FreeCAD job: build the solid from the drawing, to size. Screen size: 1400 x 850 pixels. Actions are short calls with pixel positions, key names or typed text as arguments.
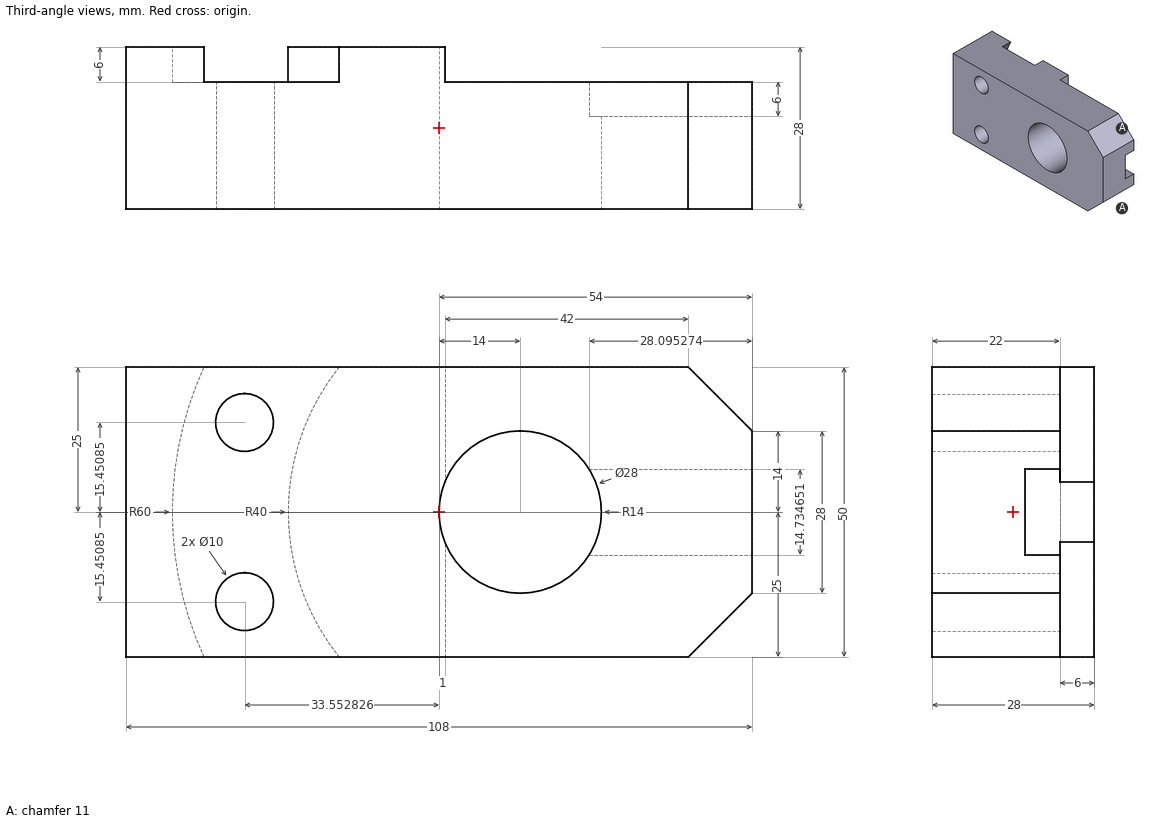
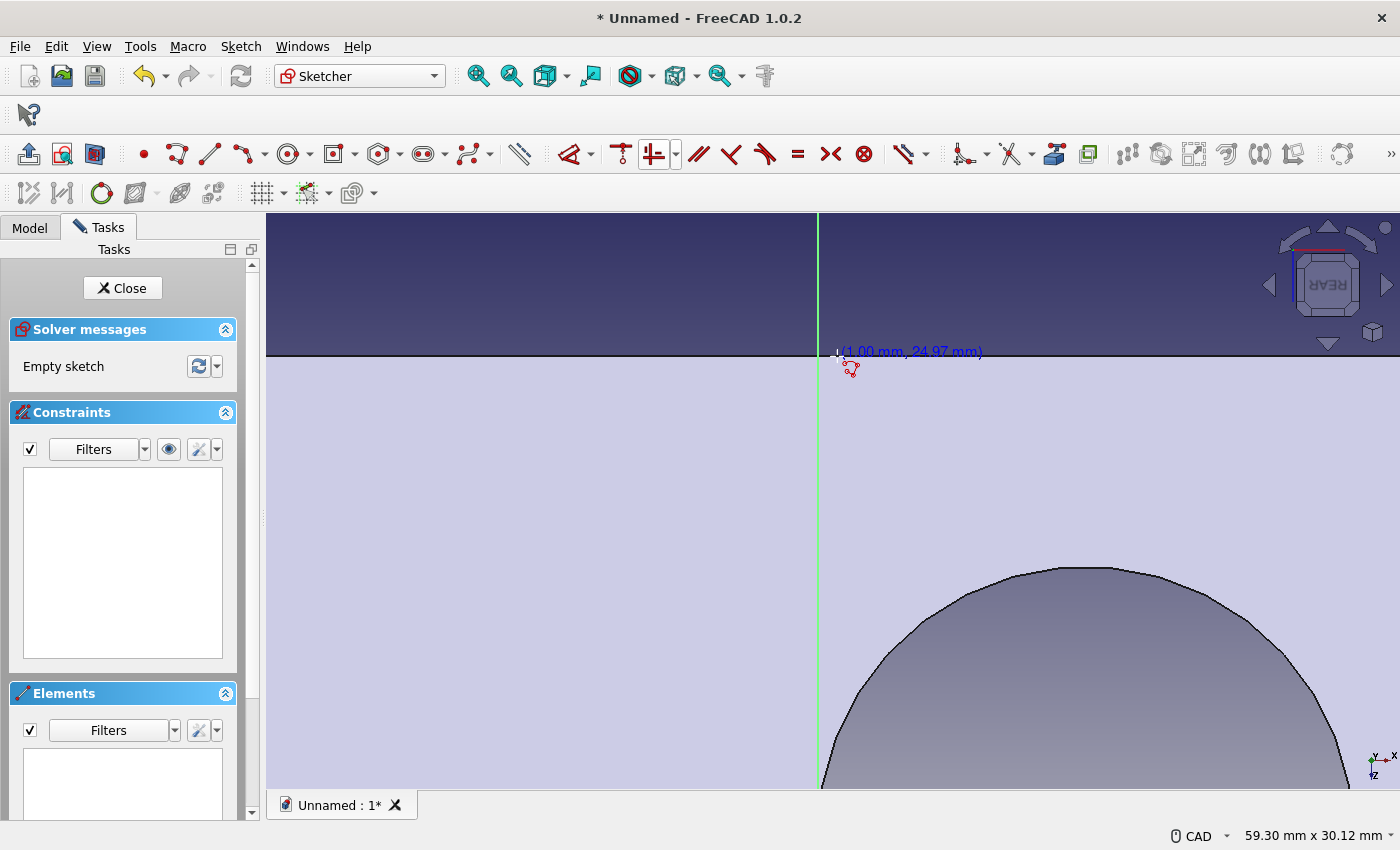
scroll(433, 307, down, 5)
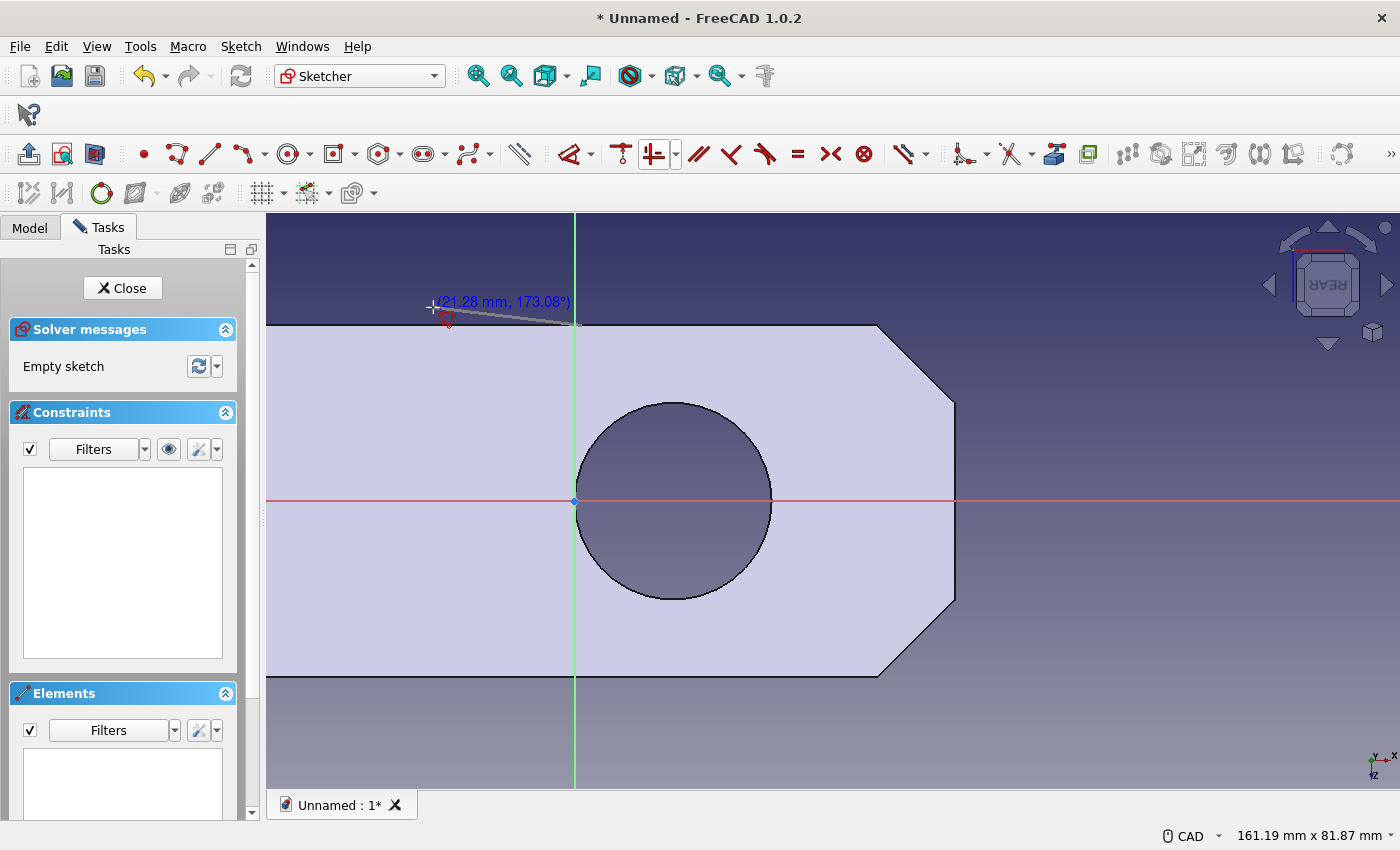
scroll(582, 677, up, 5)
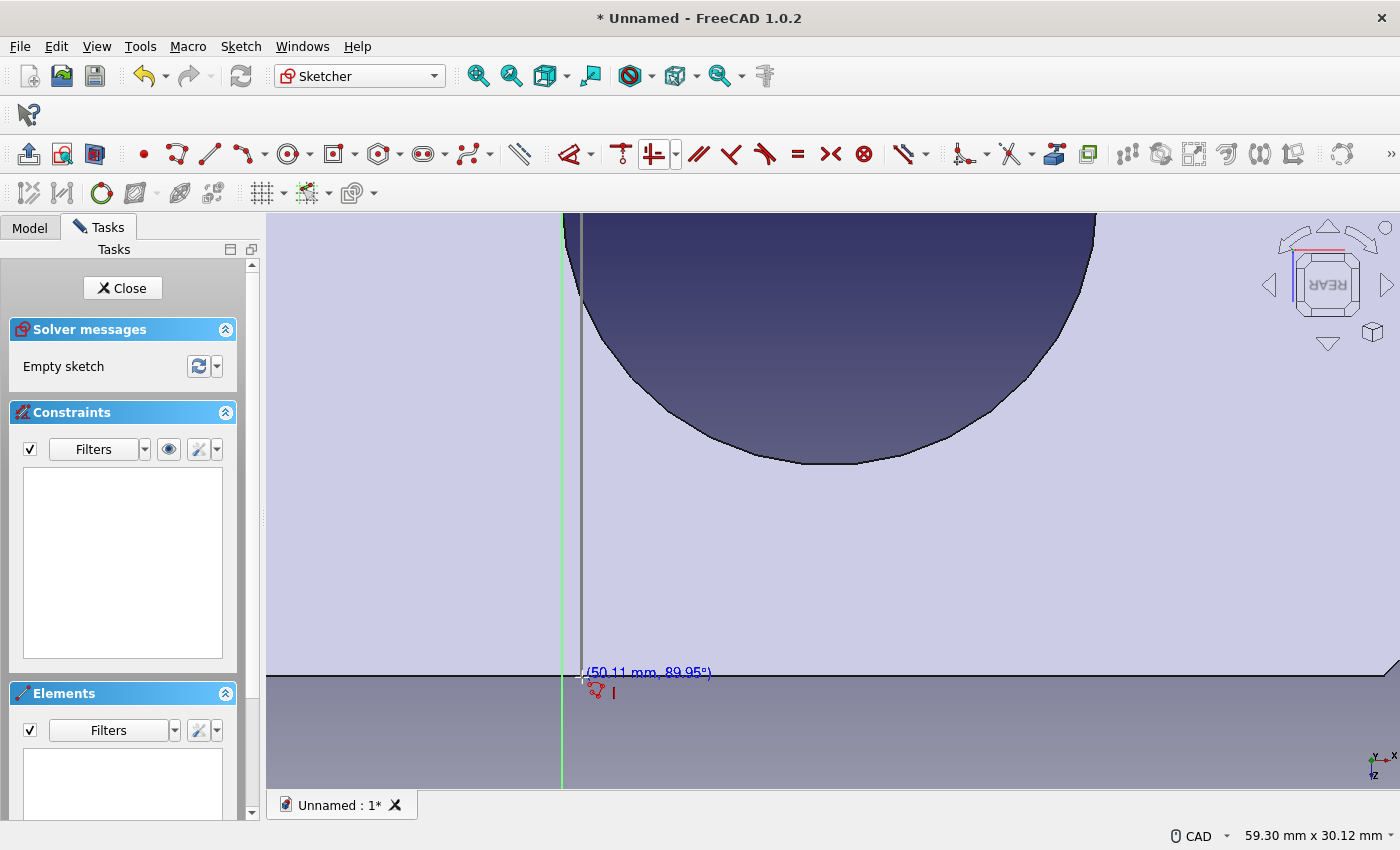
click(581, 676)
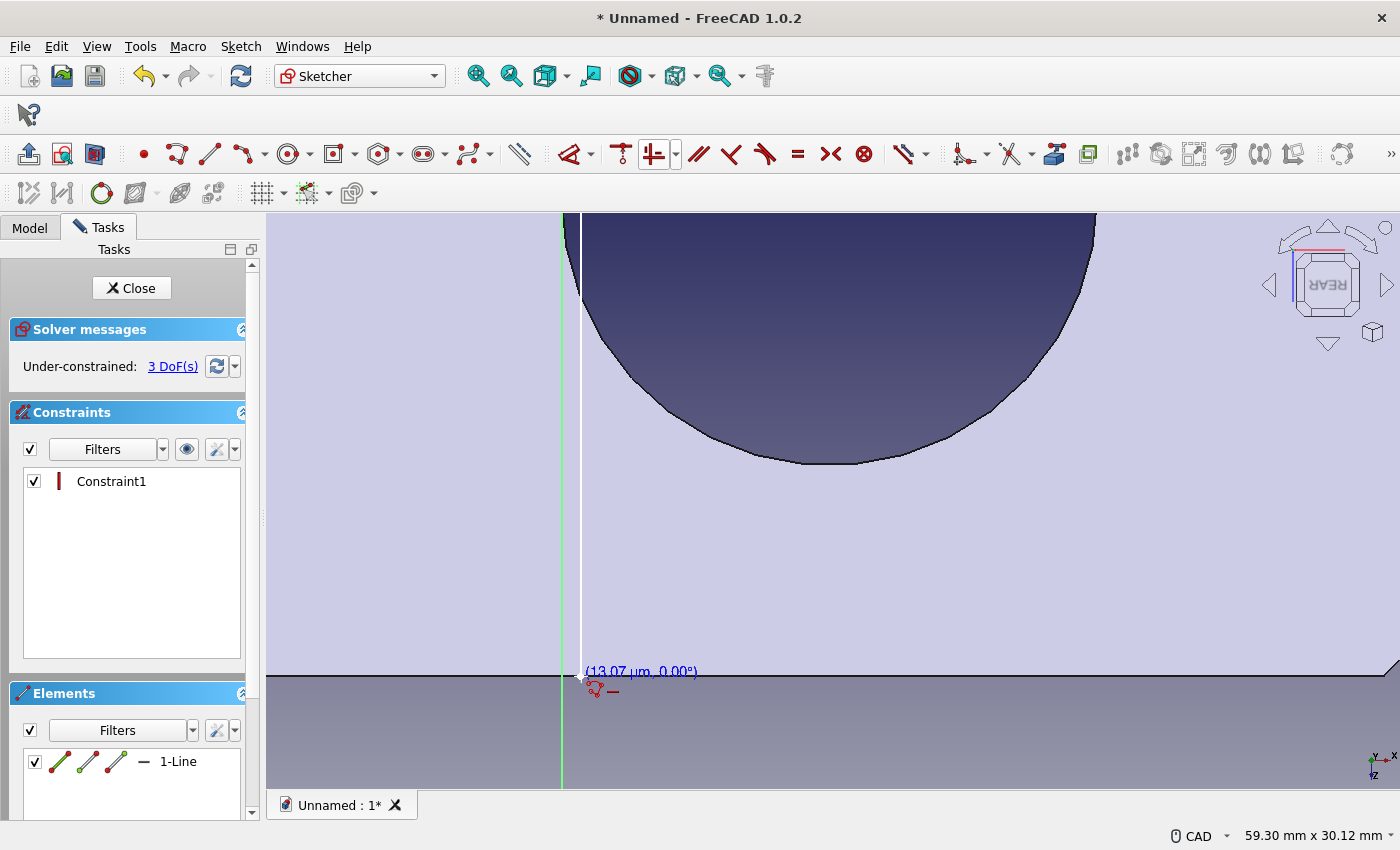
scroll(582, 678, down, 5)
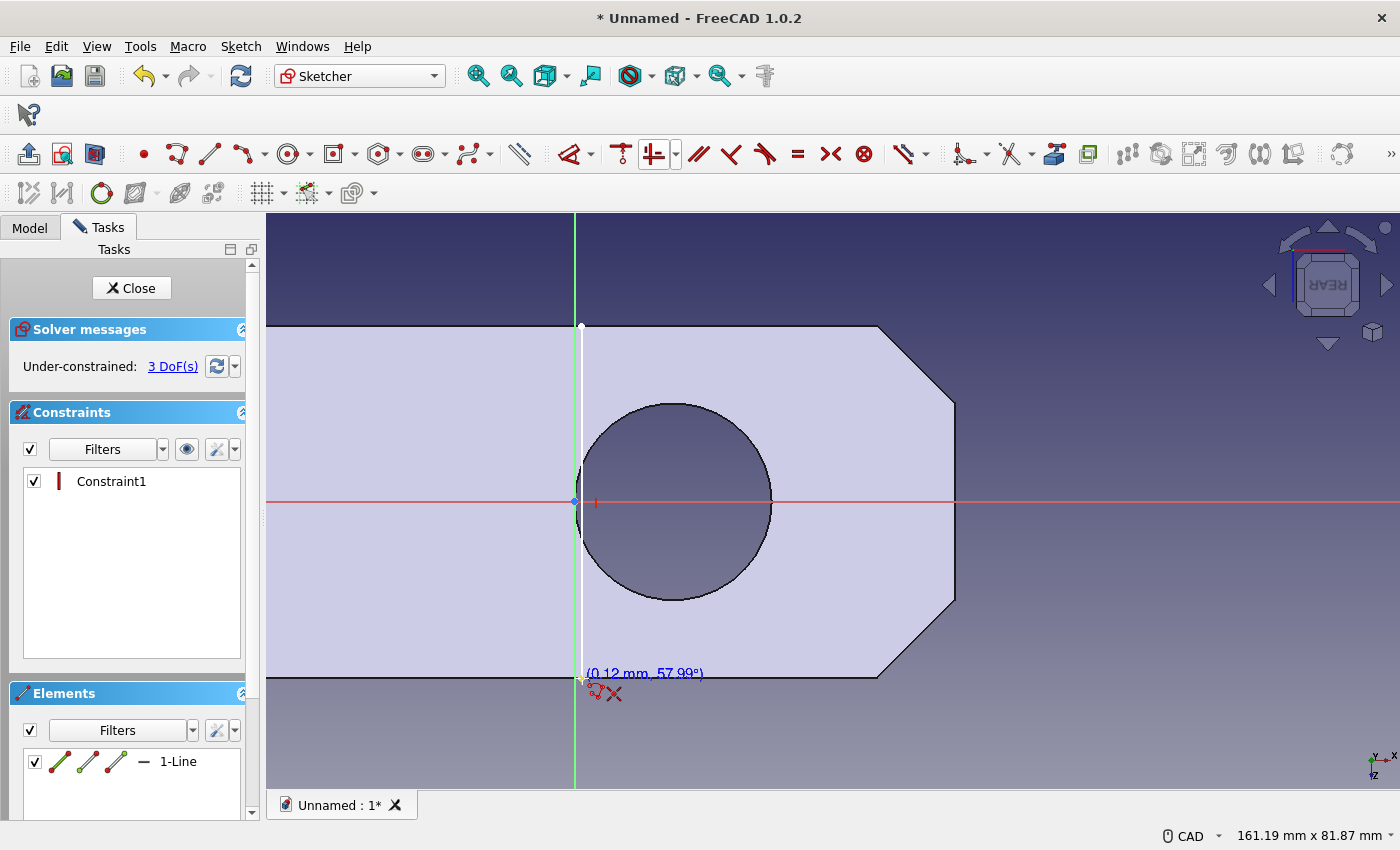
click(877, 678)
click(955, 600)
click(955, 403)
click(877, 326)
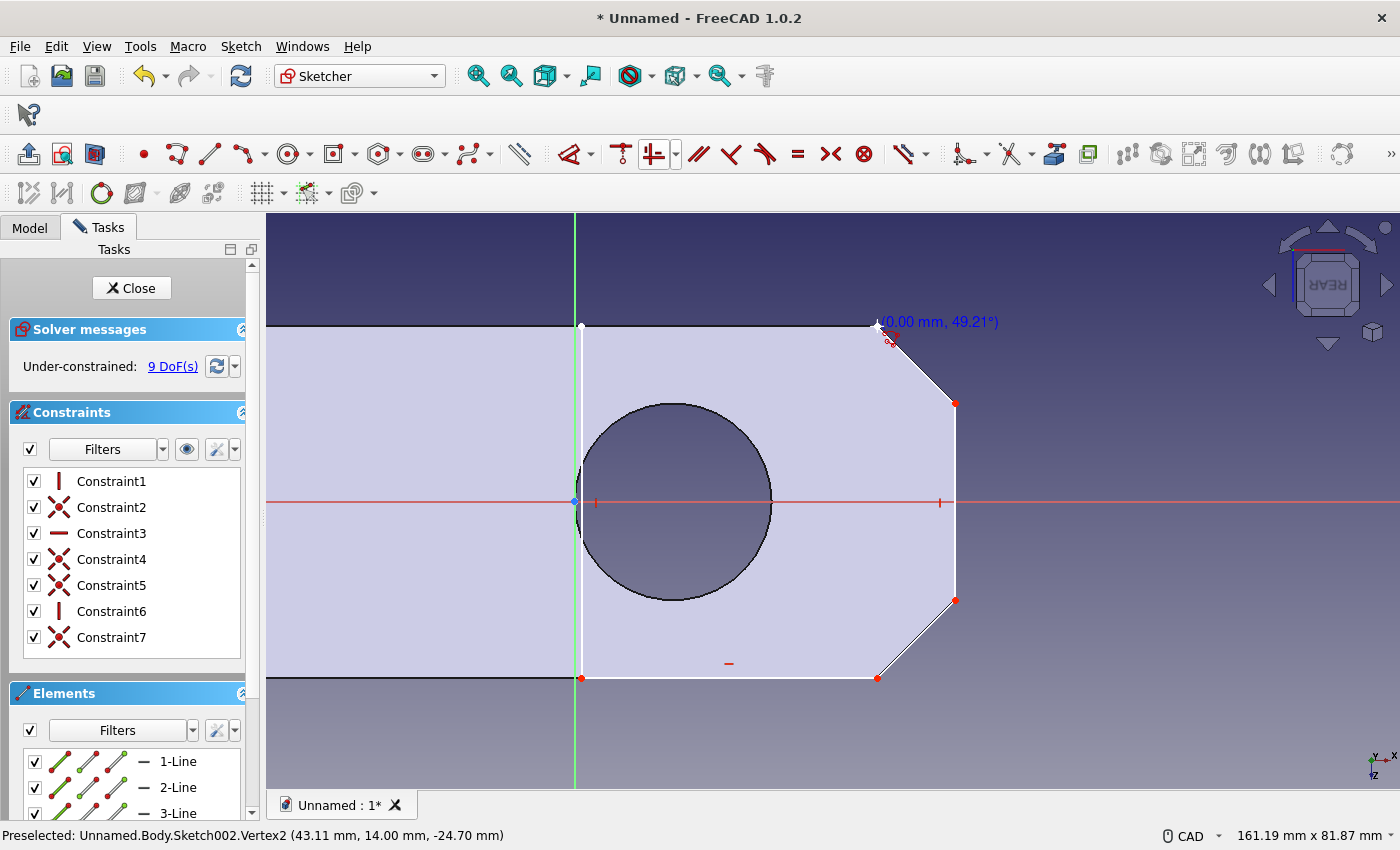
scroll(582, 326, up, 5)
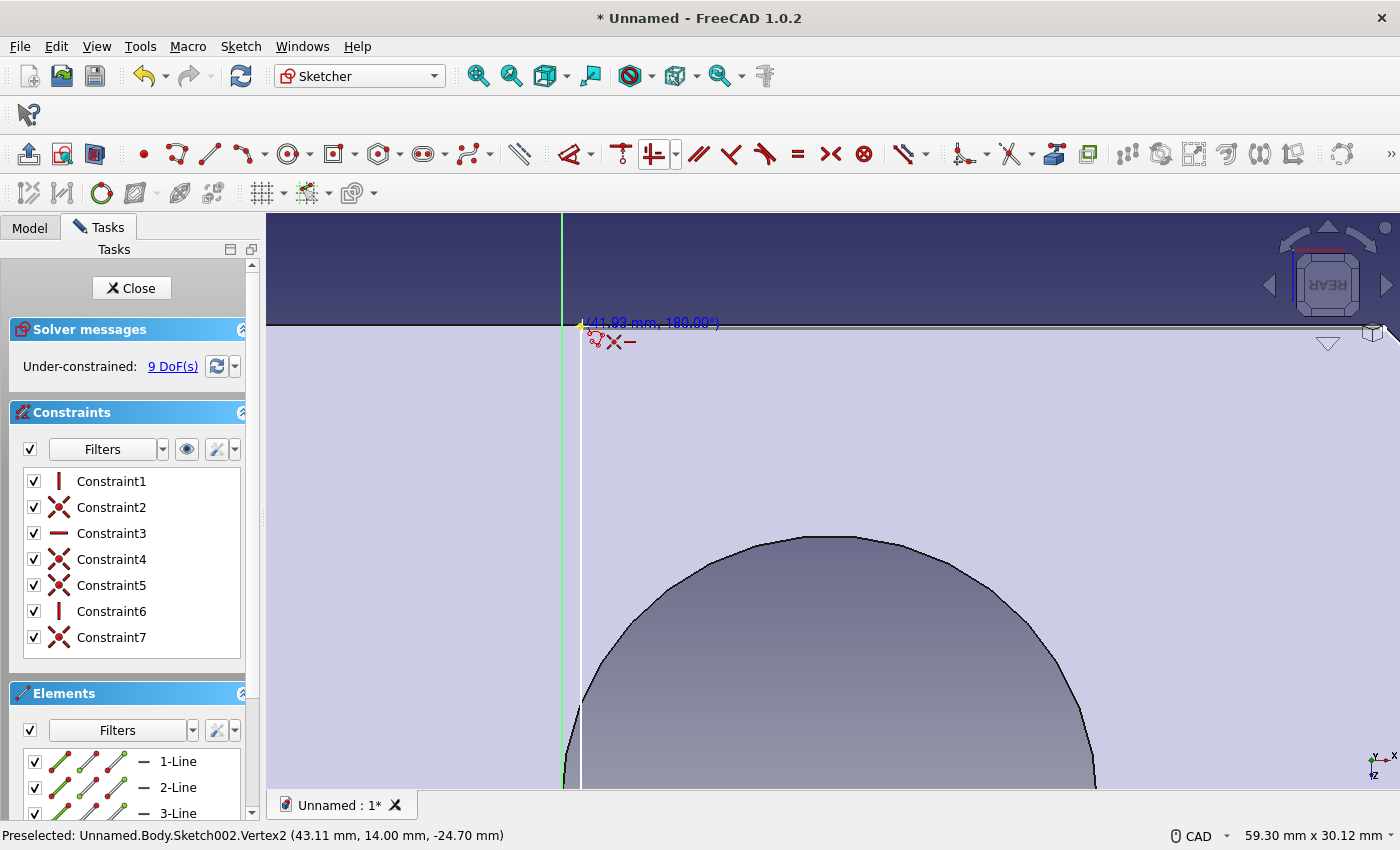
click(581, 326)
key(Escape)
key(Escape)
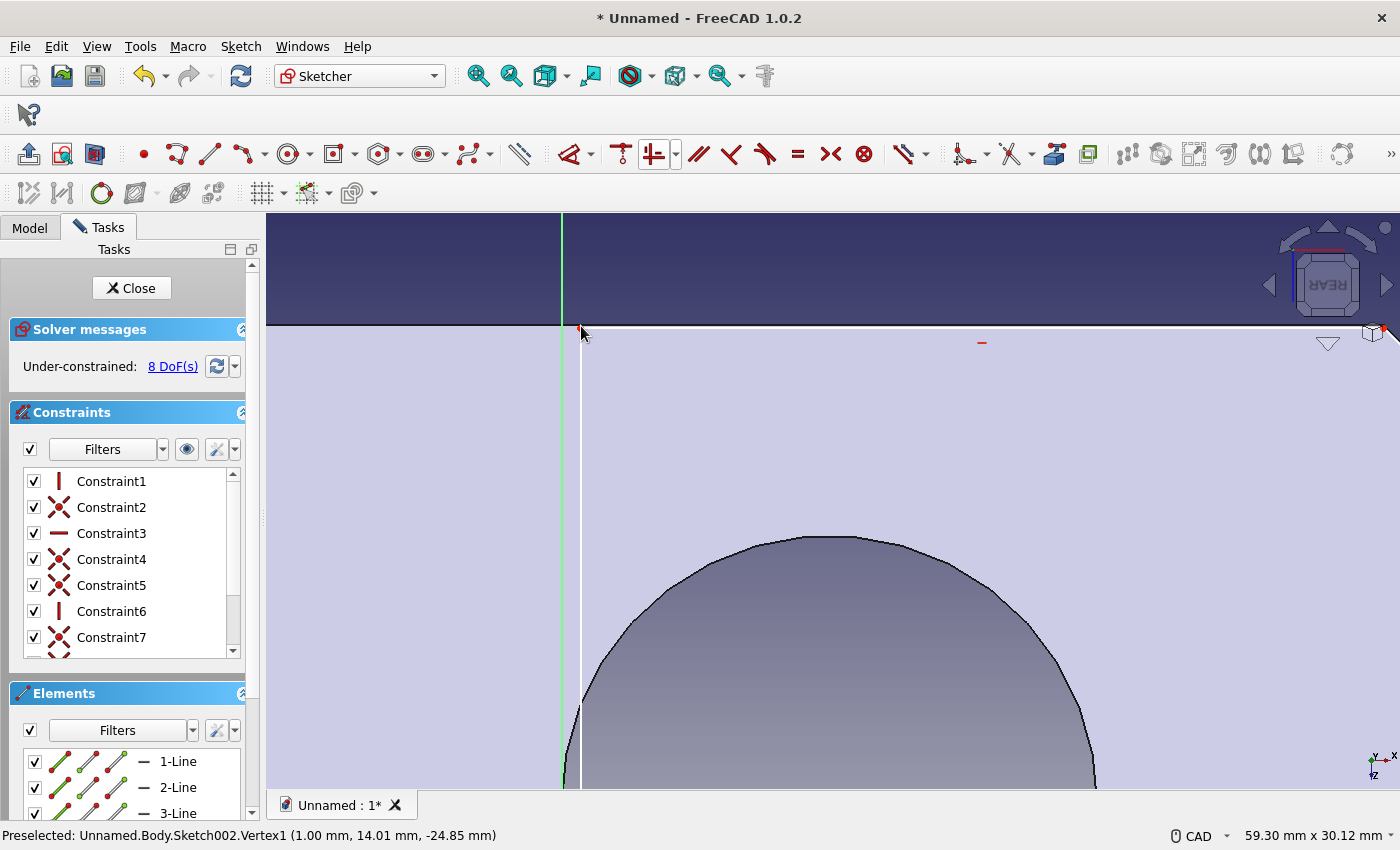
click(568, 154)